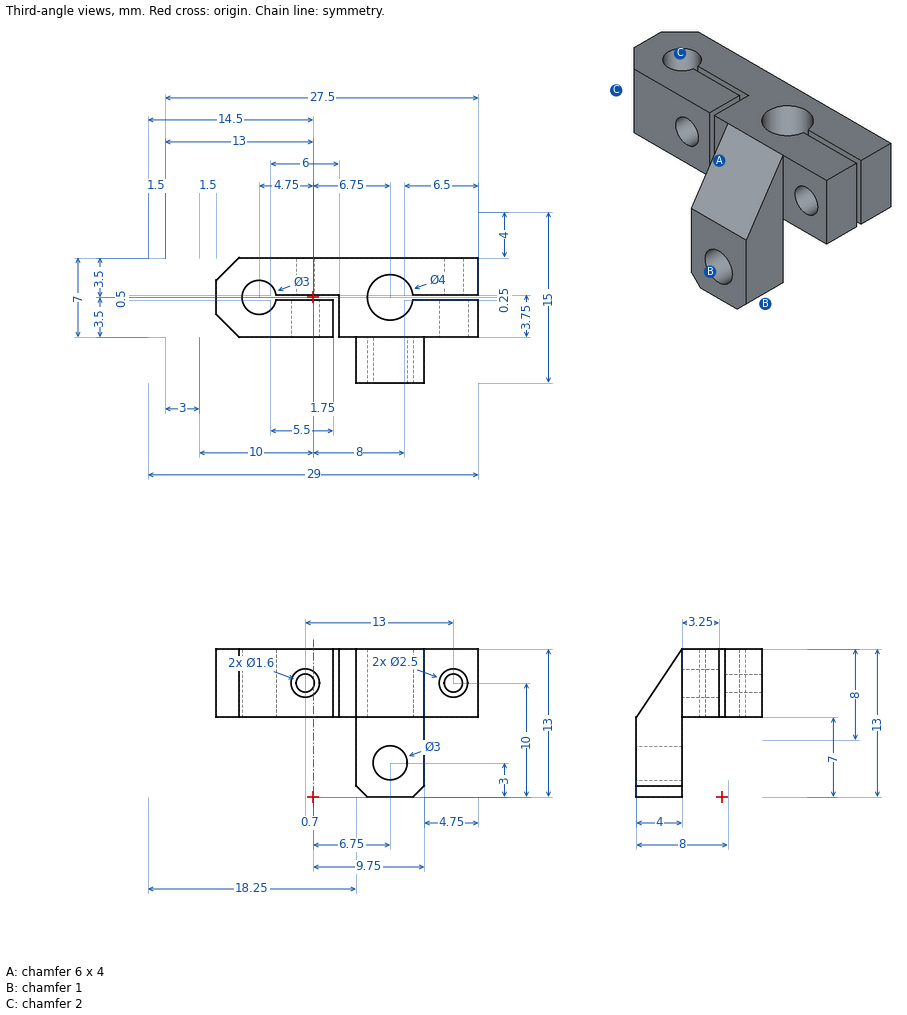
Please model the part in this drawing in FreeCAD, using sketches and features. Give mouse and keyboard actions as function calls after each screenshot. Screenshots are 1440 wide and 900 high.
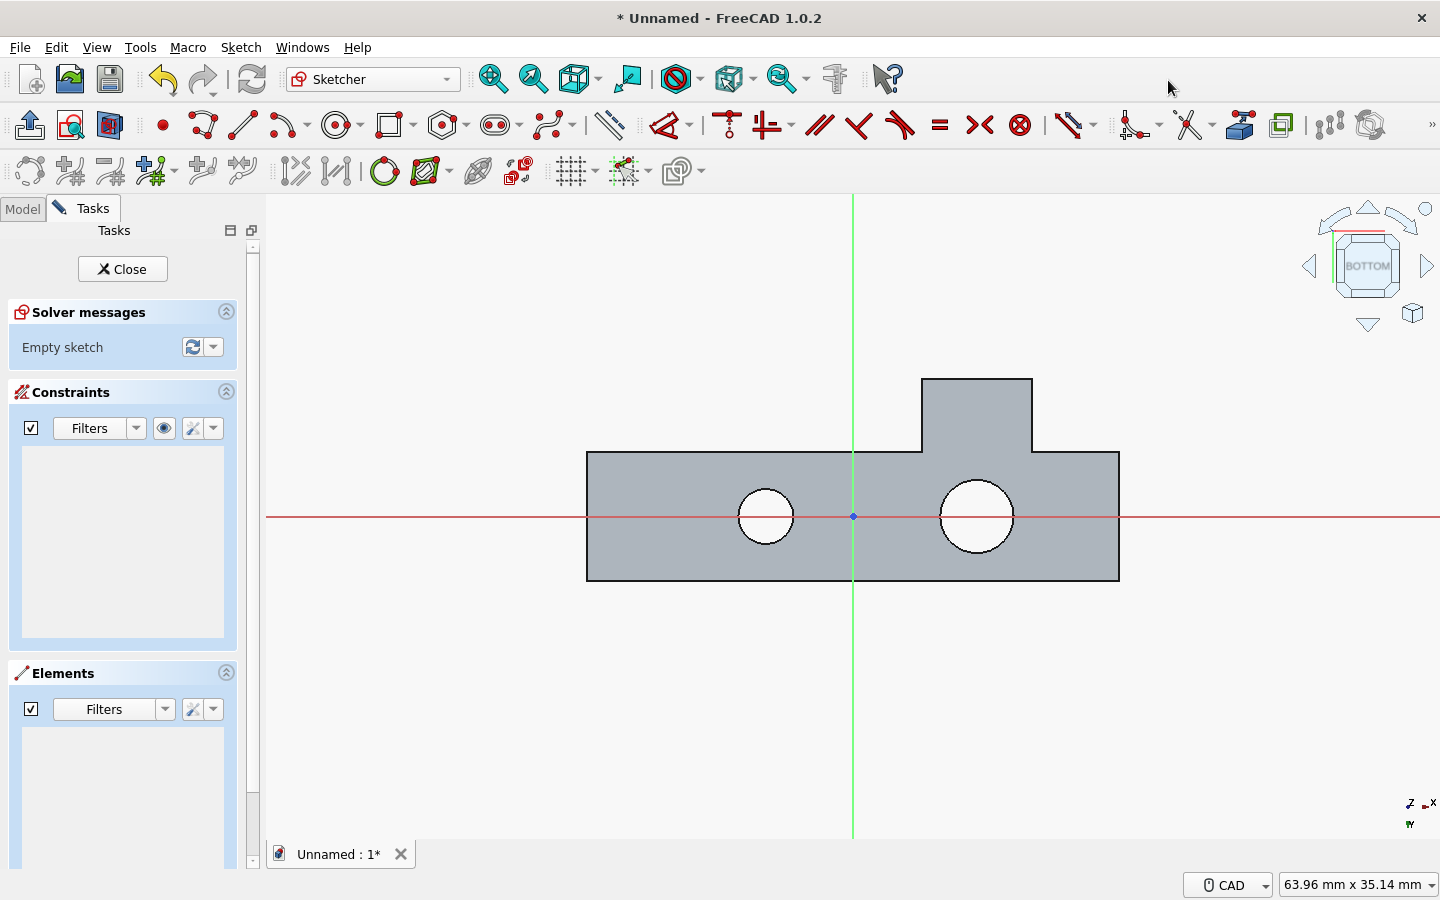
scroll(682, 517, up, 5)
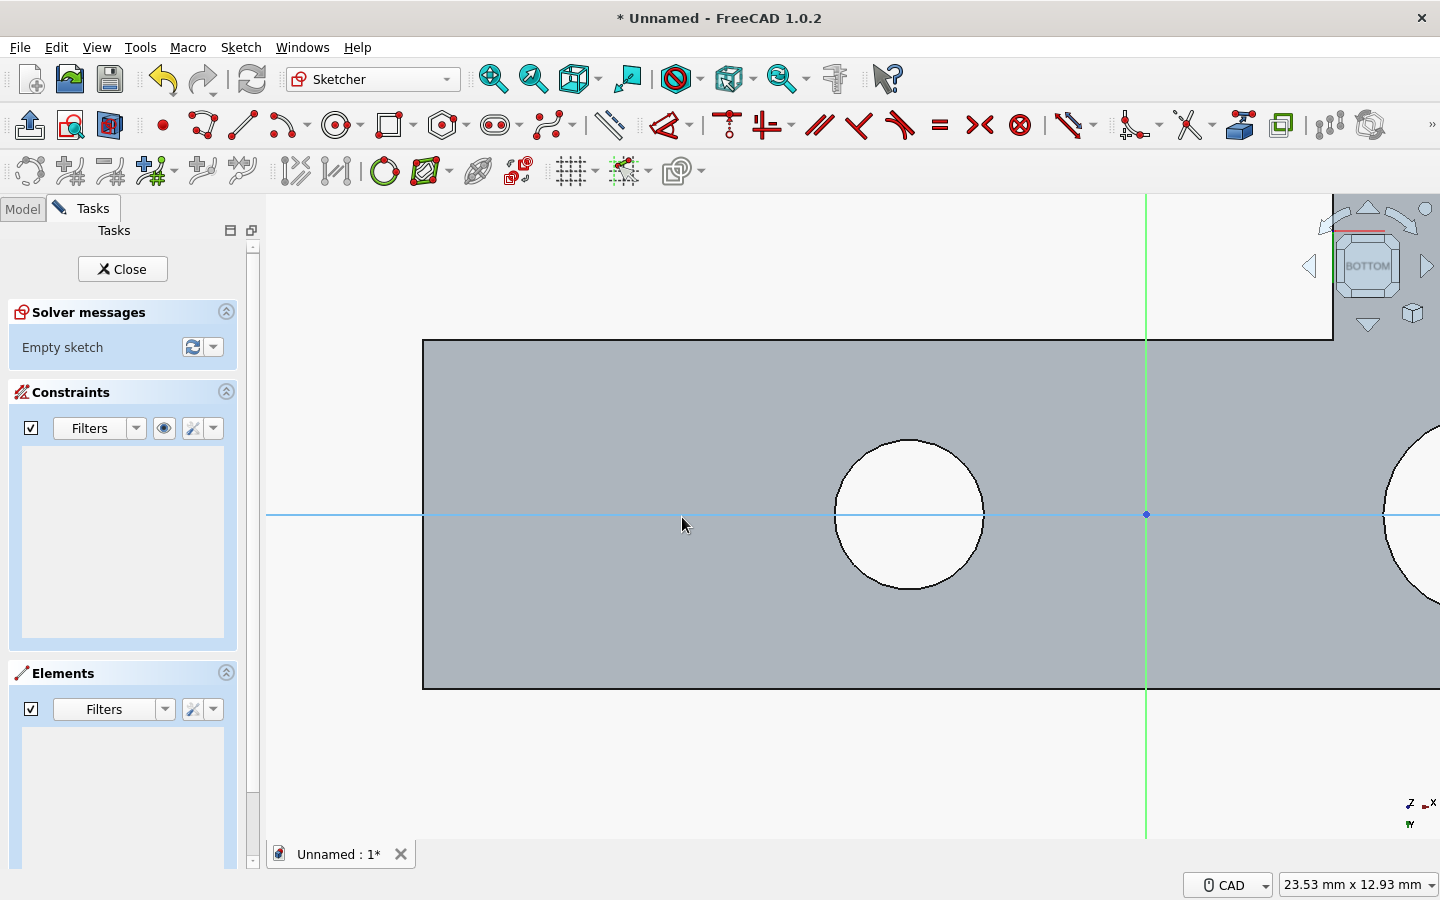
click(390, 126)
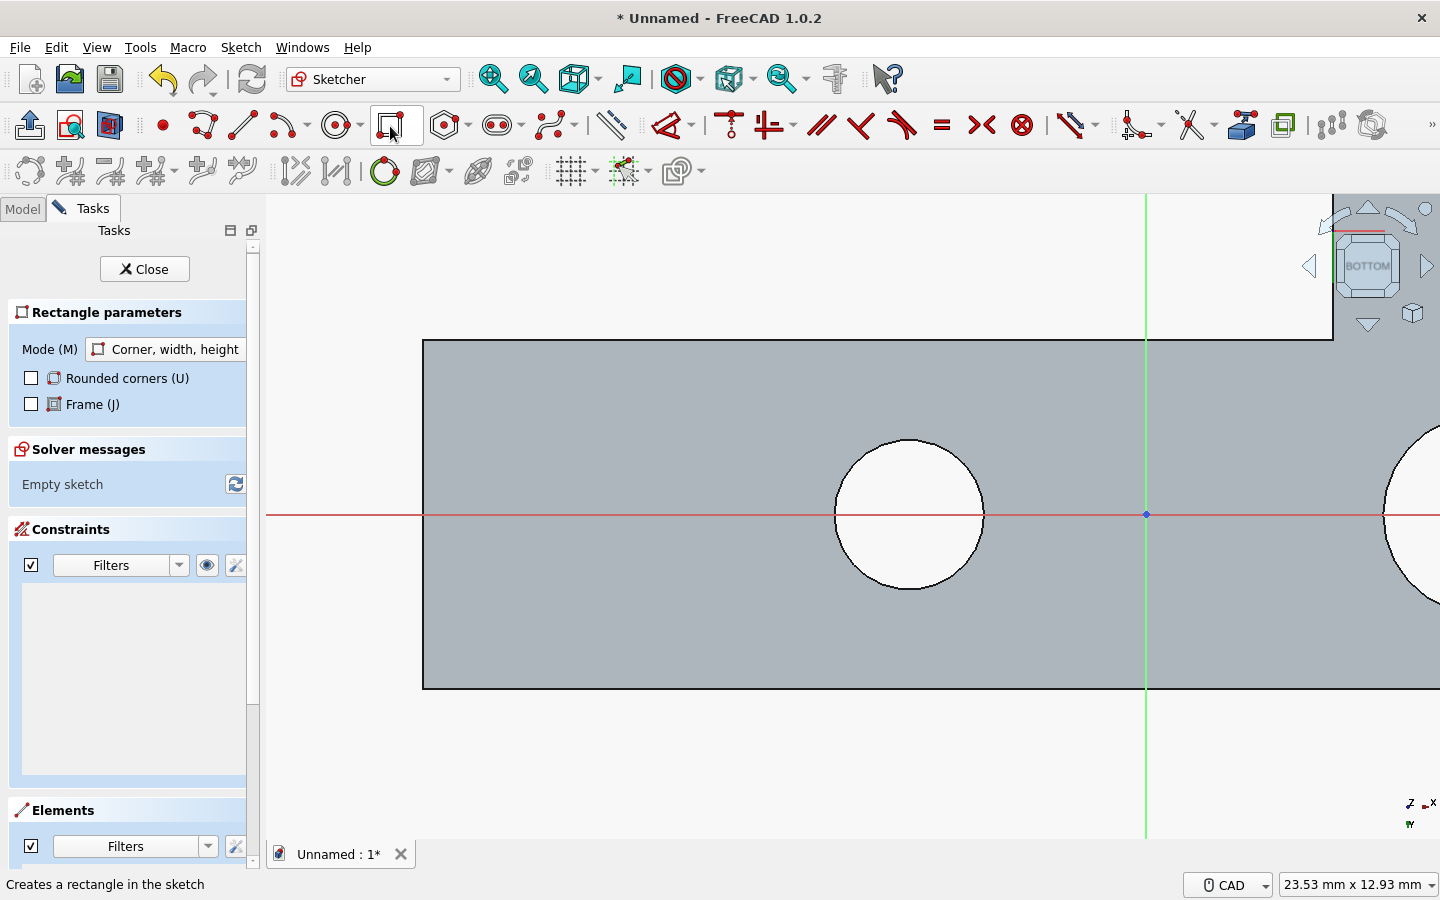
click(423, 340)
move(498, 689)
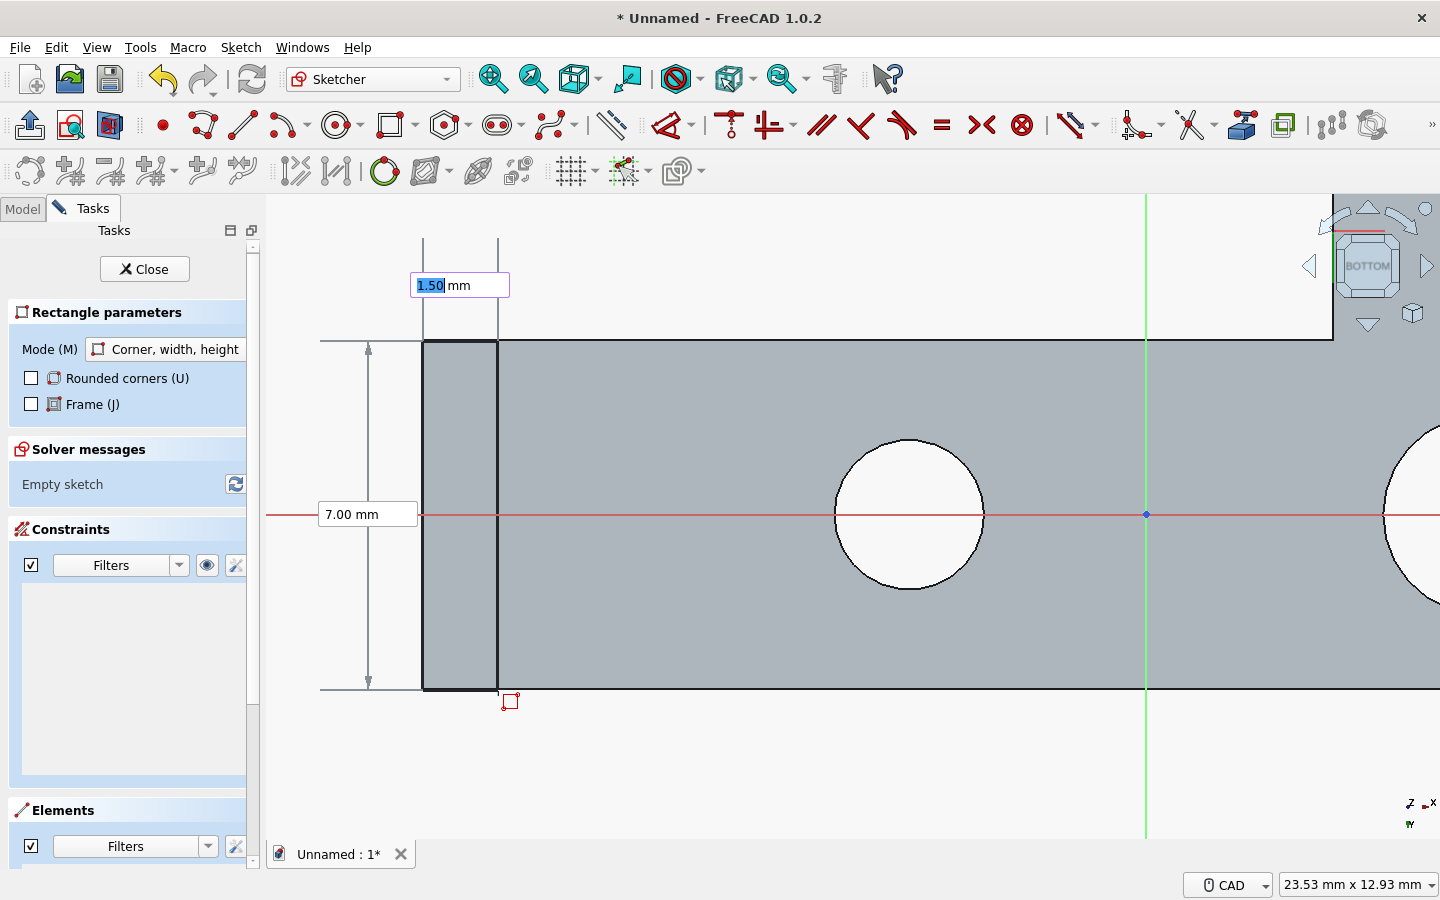
text(1.5)
key(Tab)
text(7)
key(Return)
key(Escape)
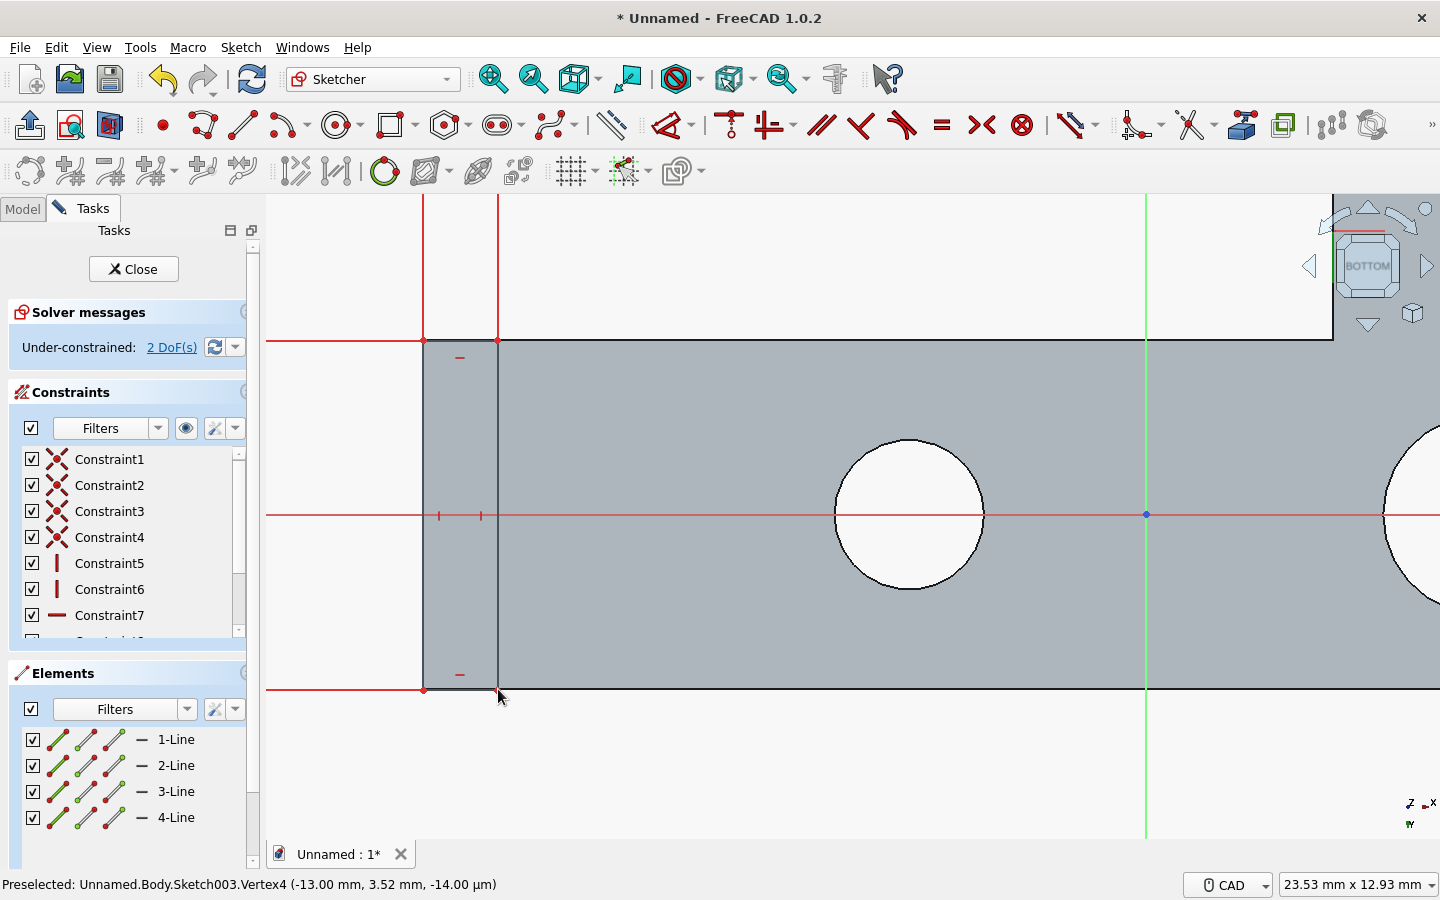
click(666, 126)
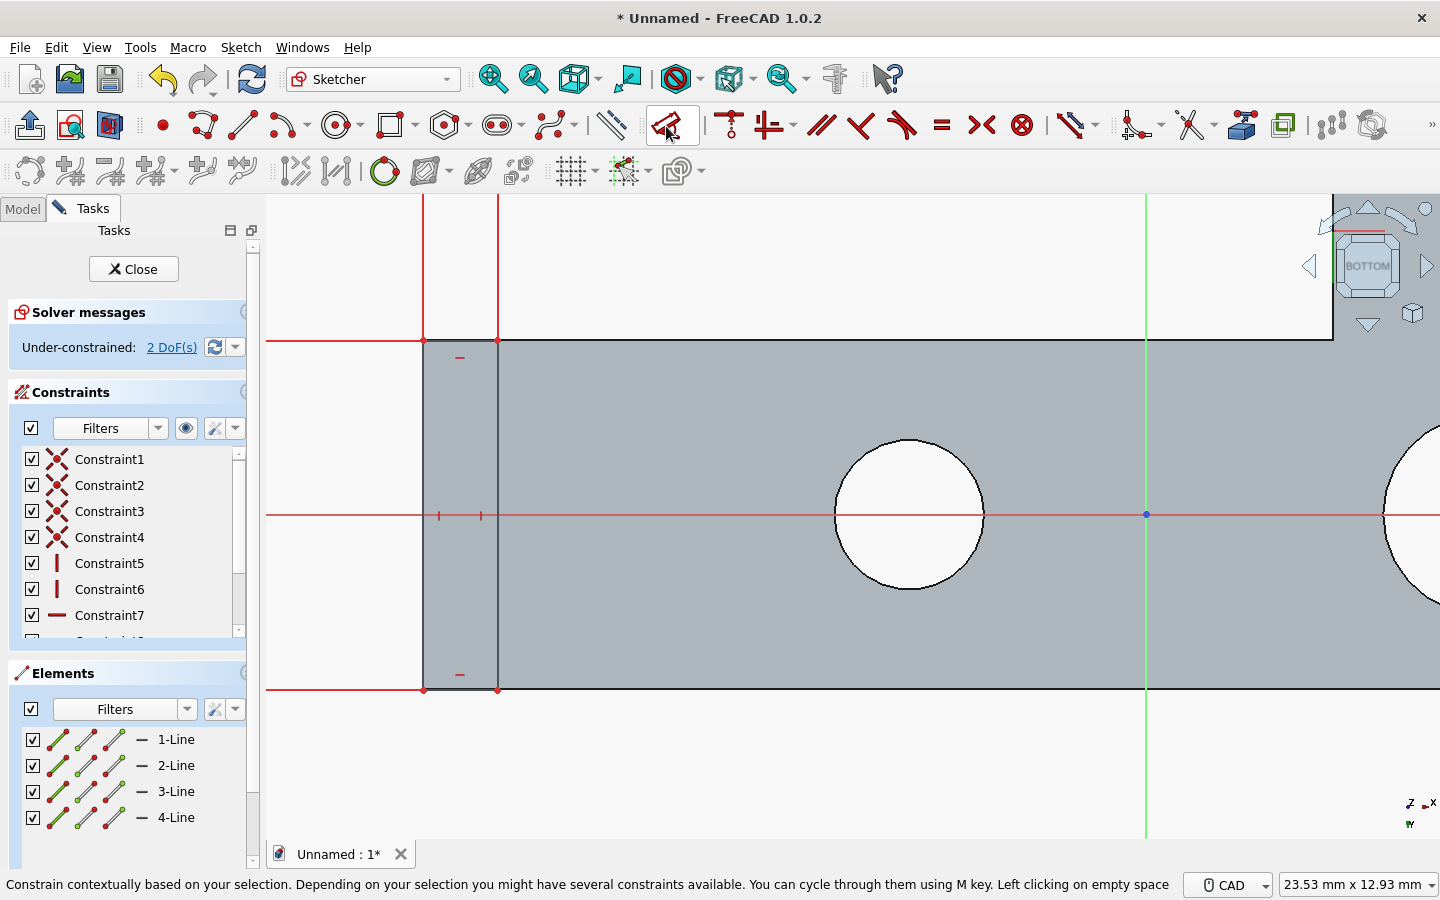
click(498, 690)
click(822, 724)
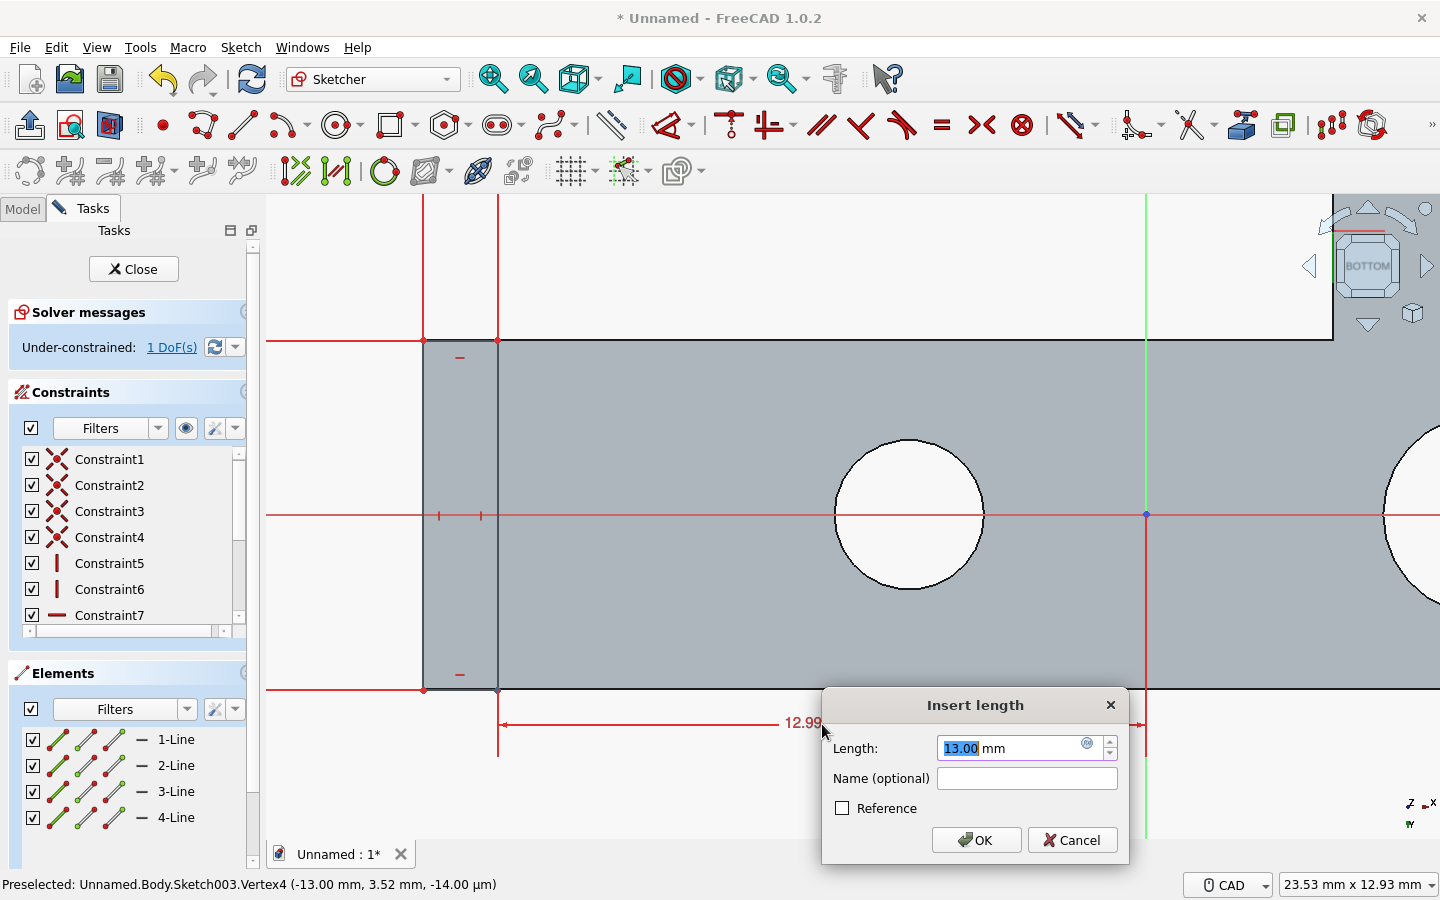
text(13)
key(Return)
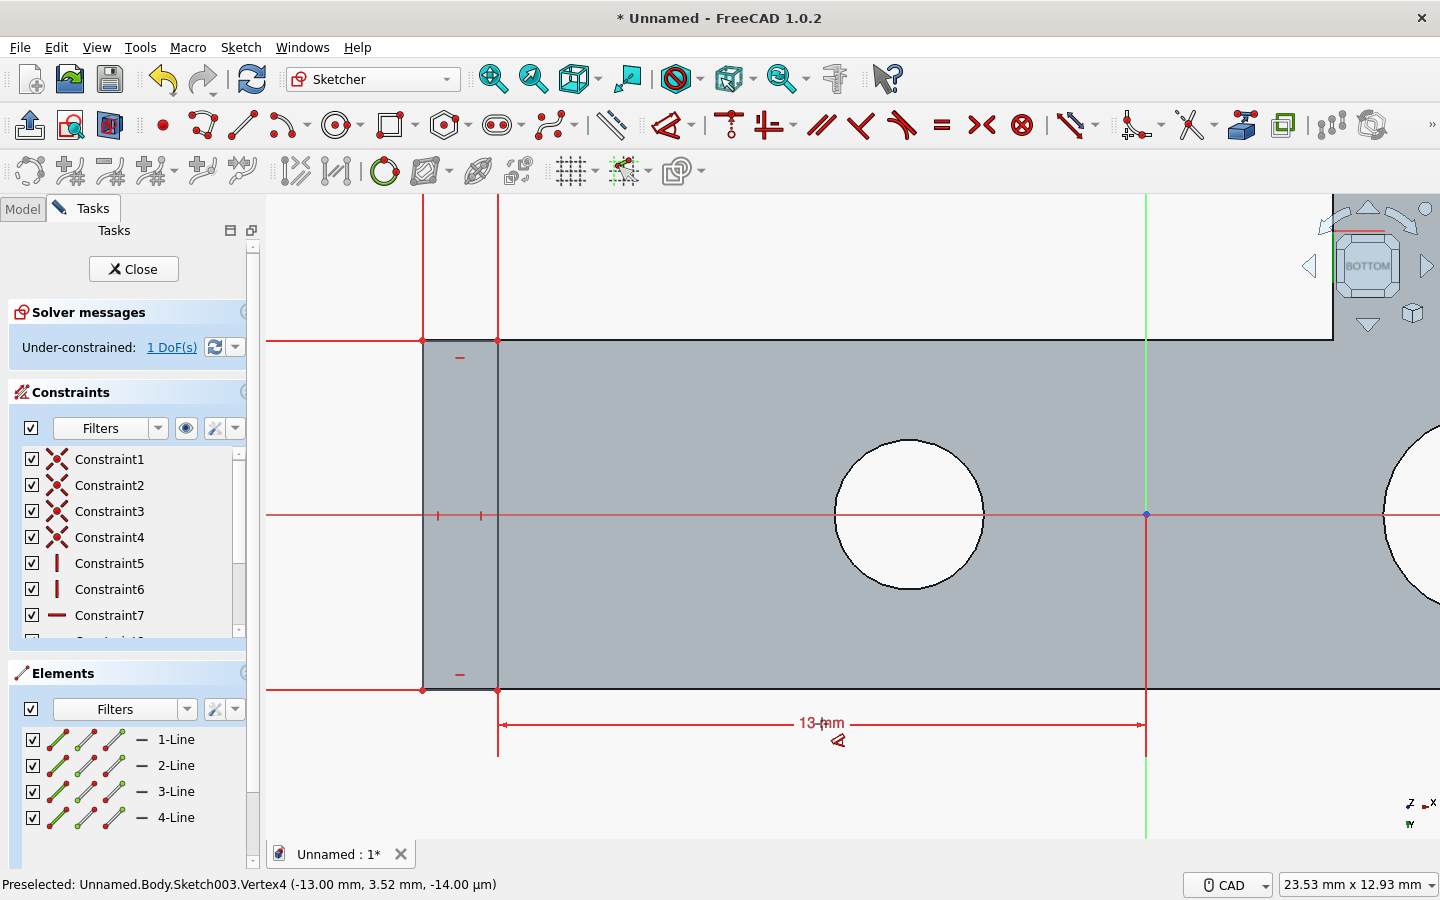
click(423, 341)
click(1180, 428)